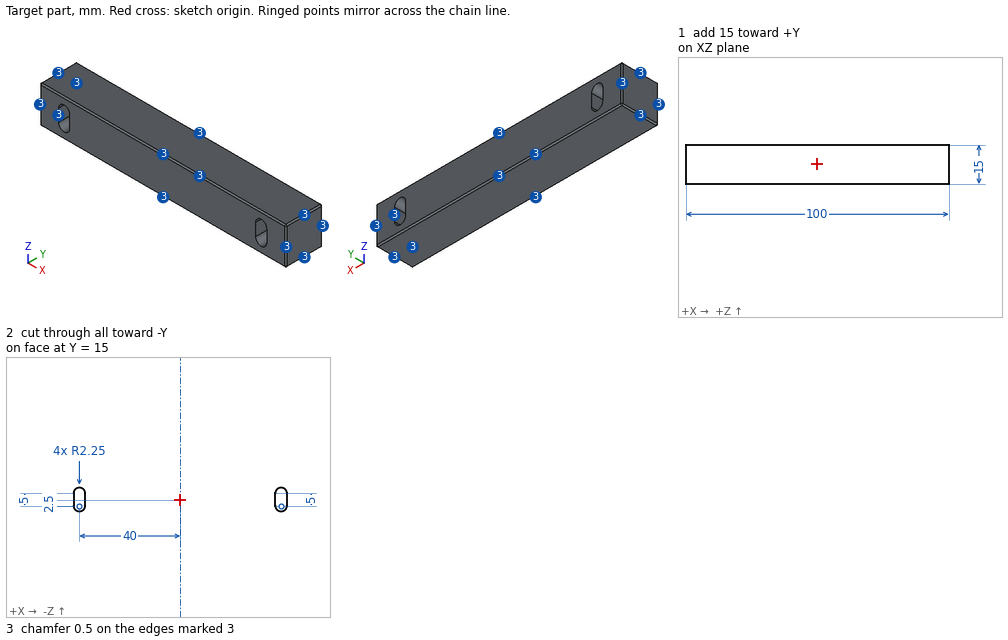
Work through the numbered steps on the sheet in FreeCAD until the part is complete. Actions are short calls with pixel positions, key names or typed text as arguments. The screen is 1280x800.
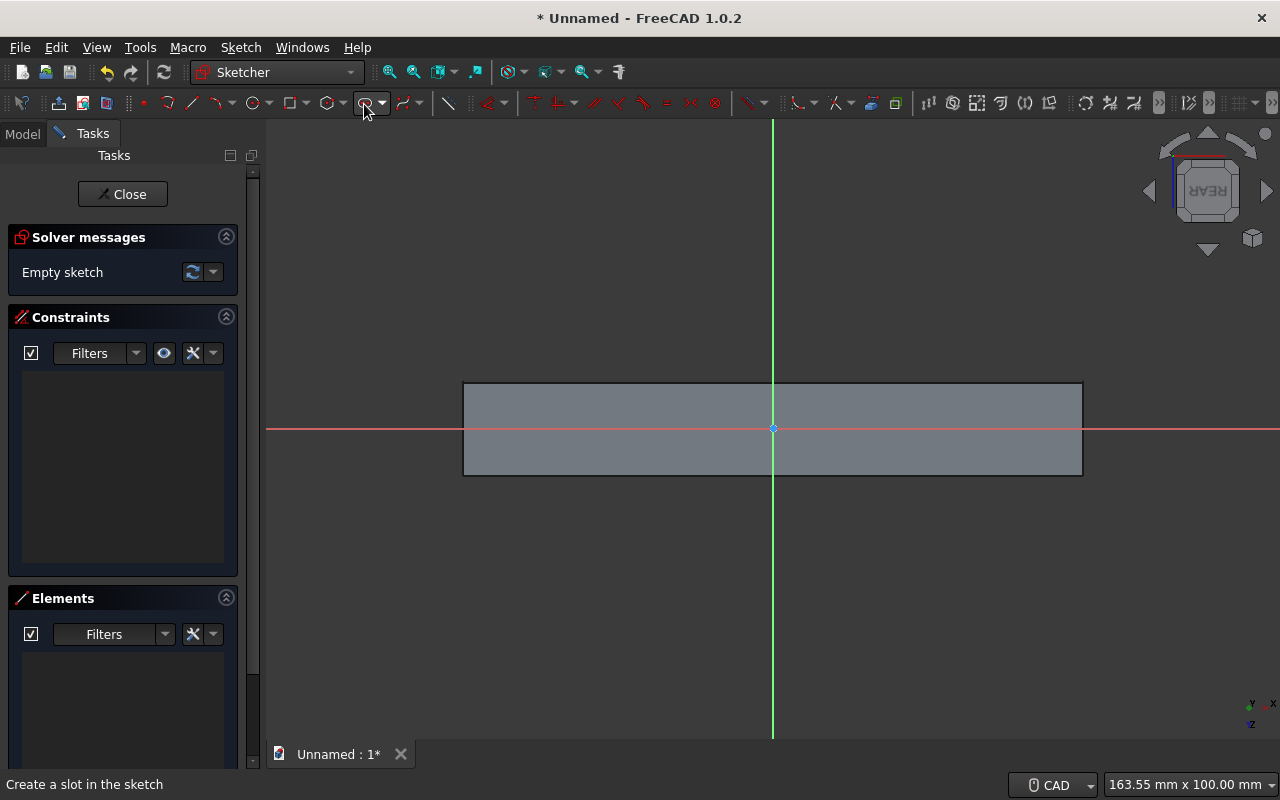
scroll(525, 445, up, 3)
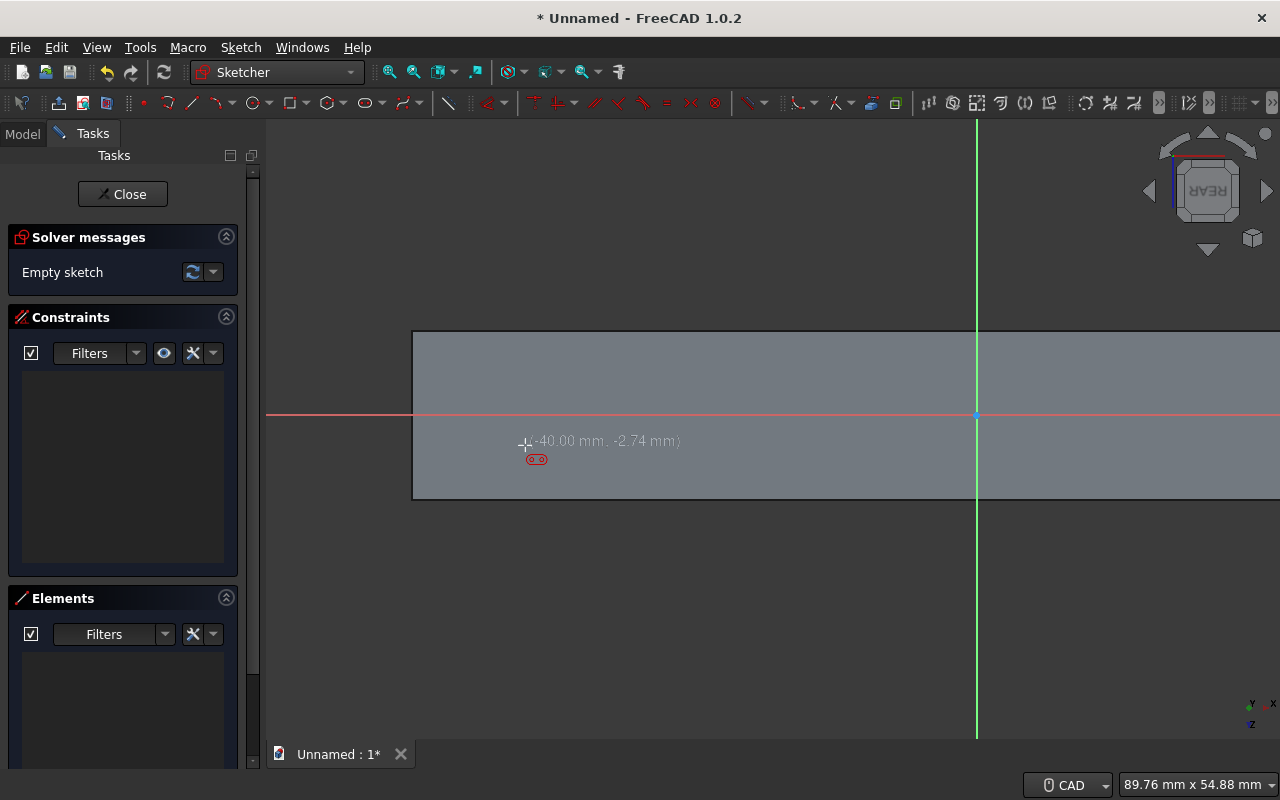
click(525, 444)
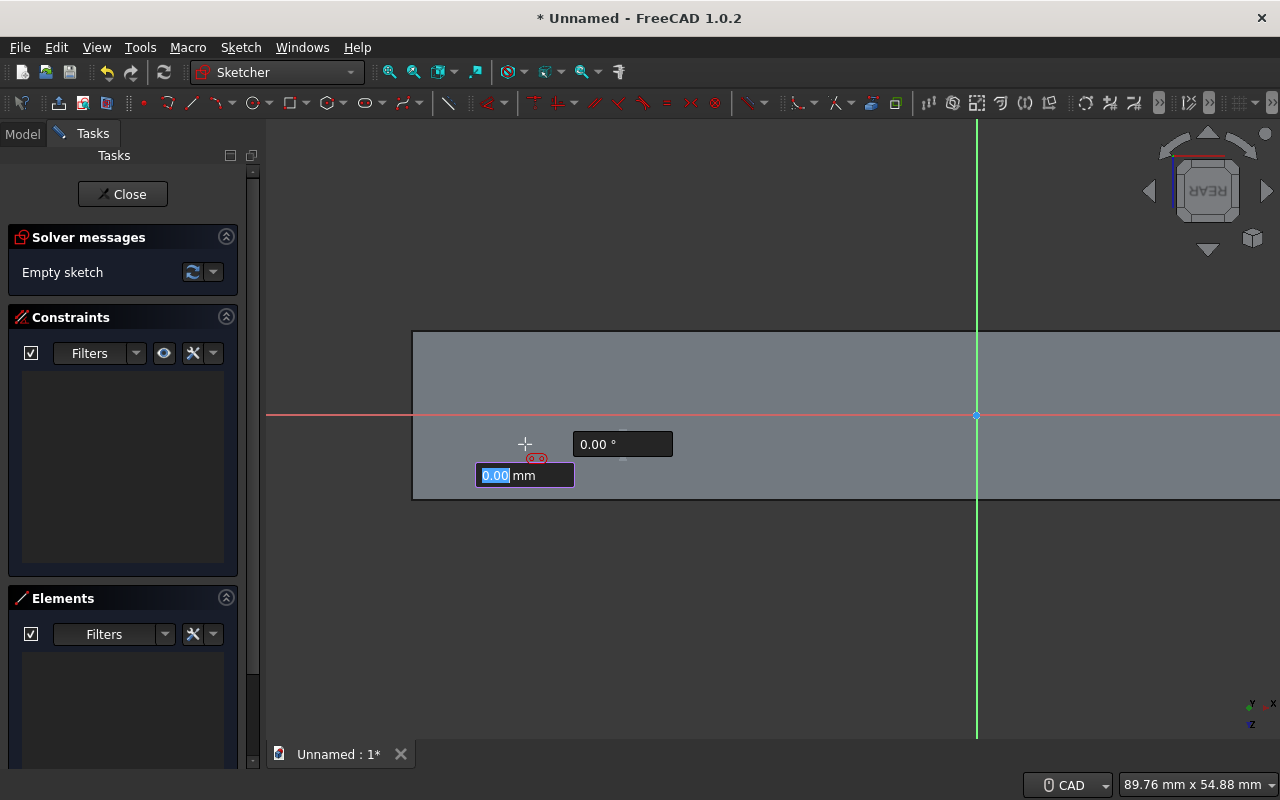
click(525, 387)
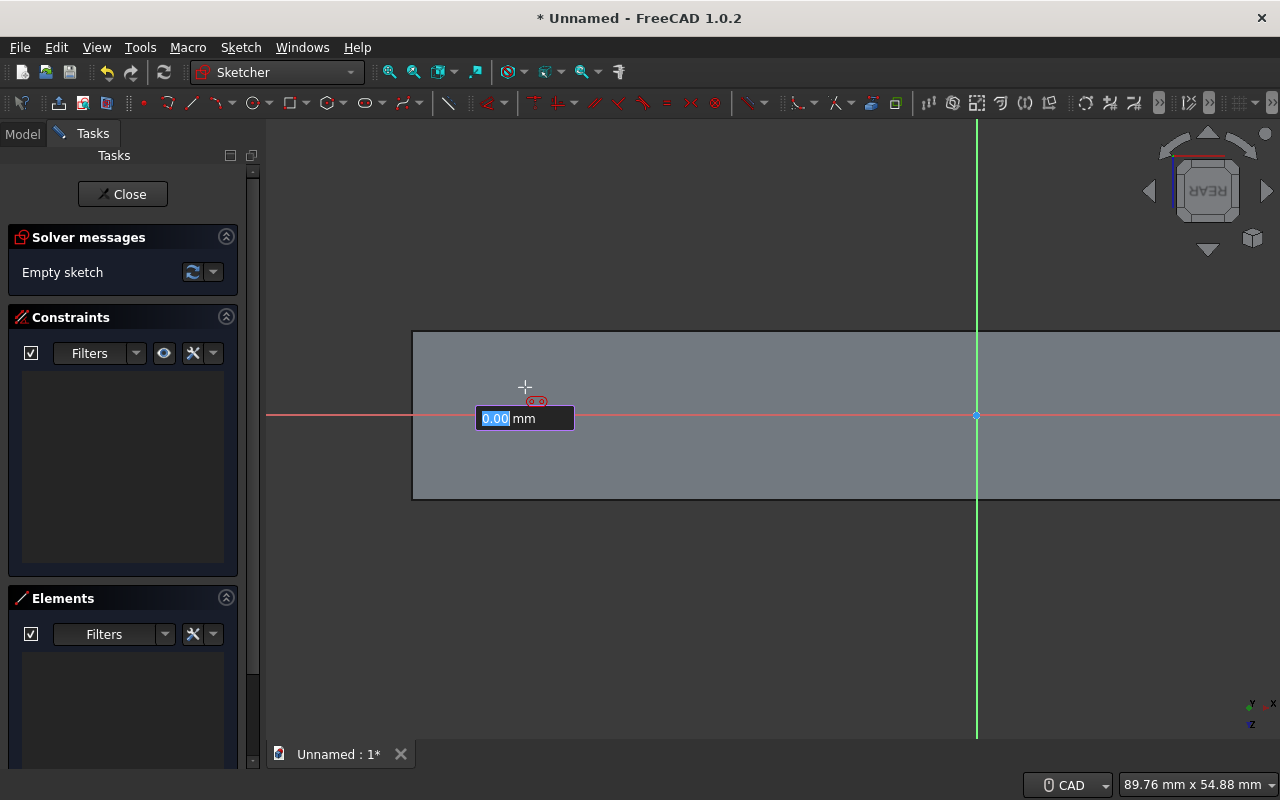
scroll(499, 407, up, 4)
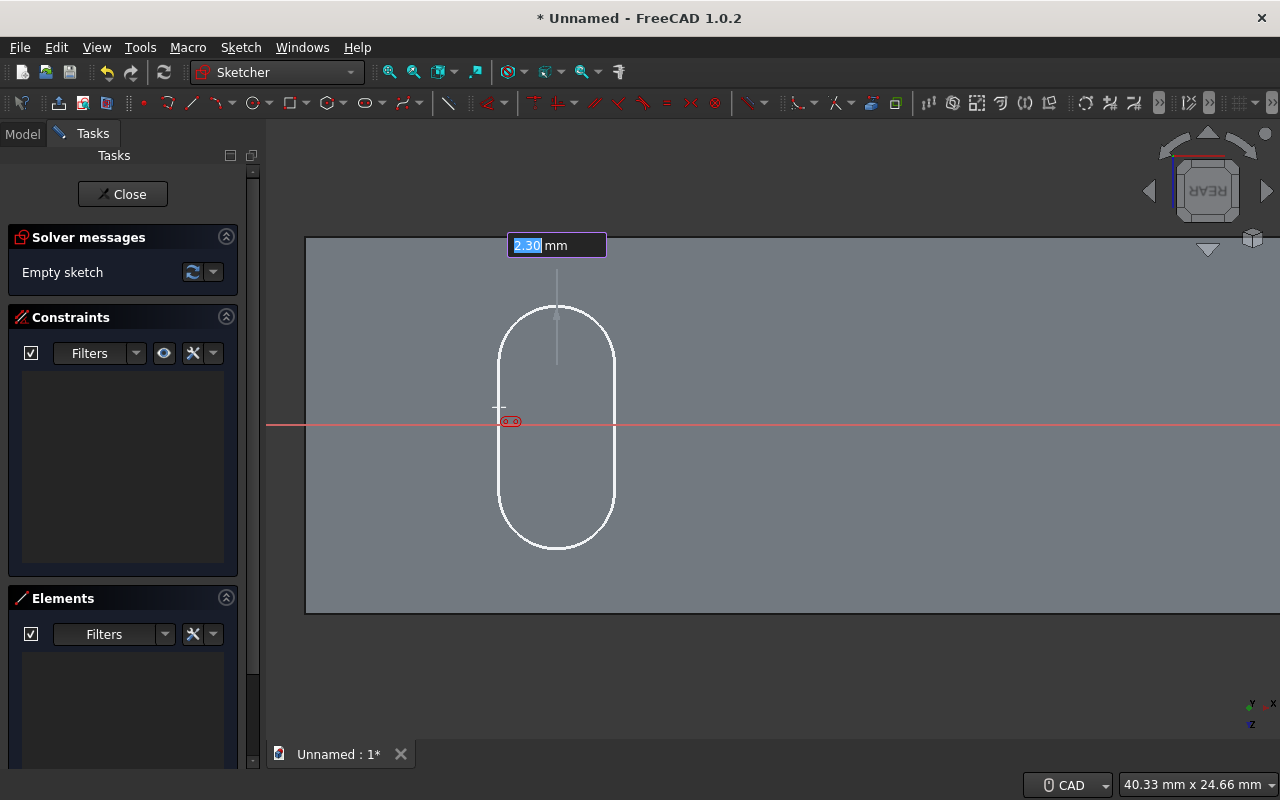
click(500, 406)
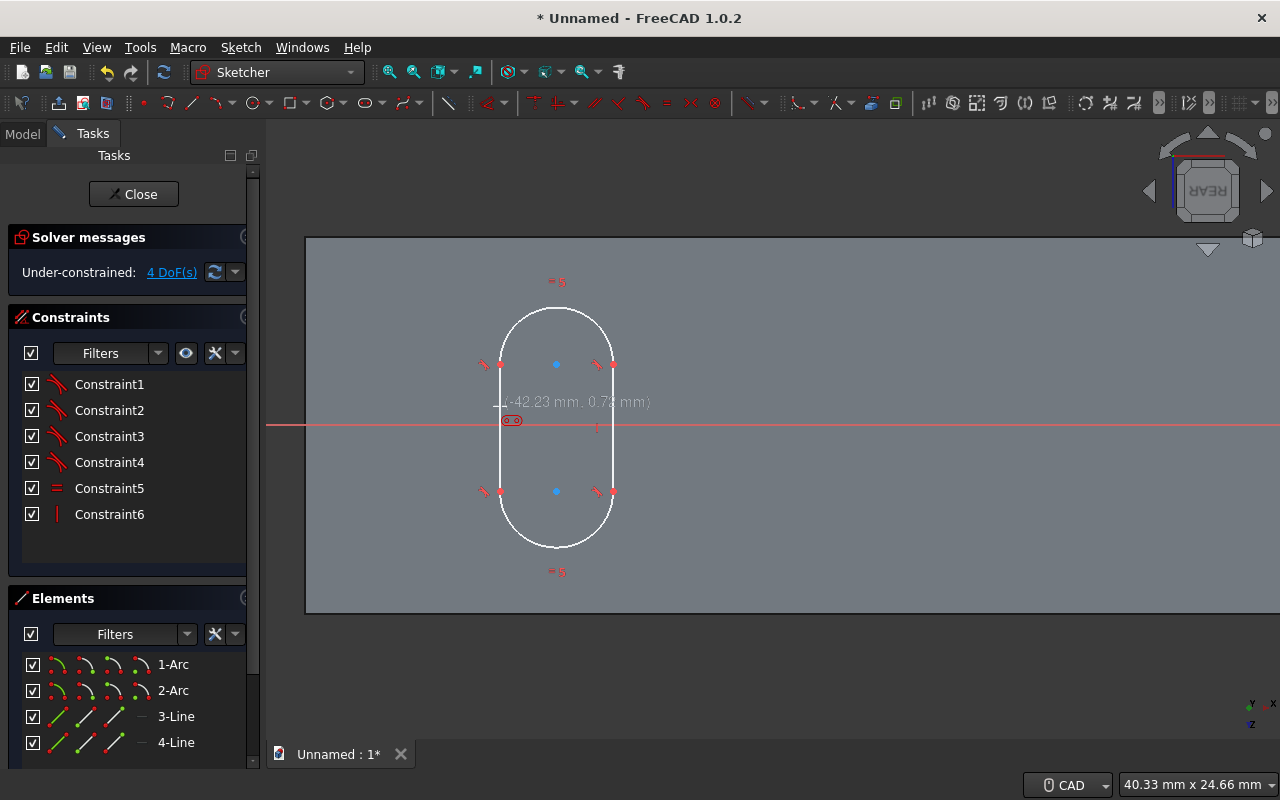
scroll(335, 431, down, 6)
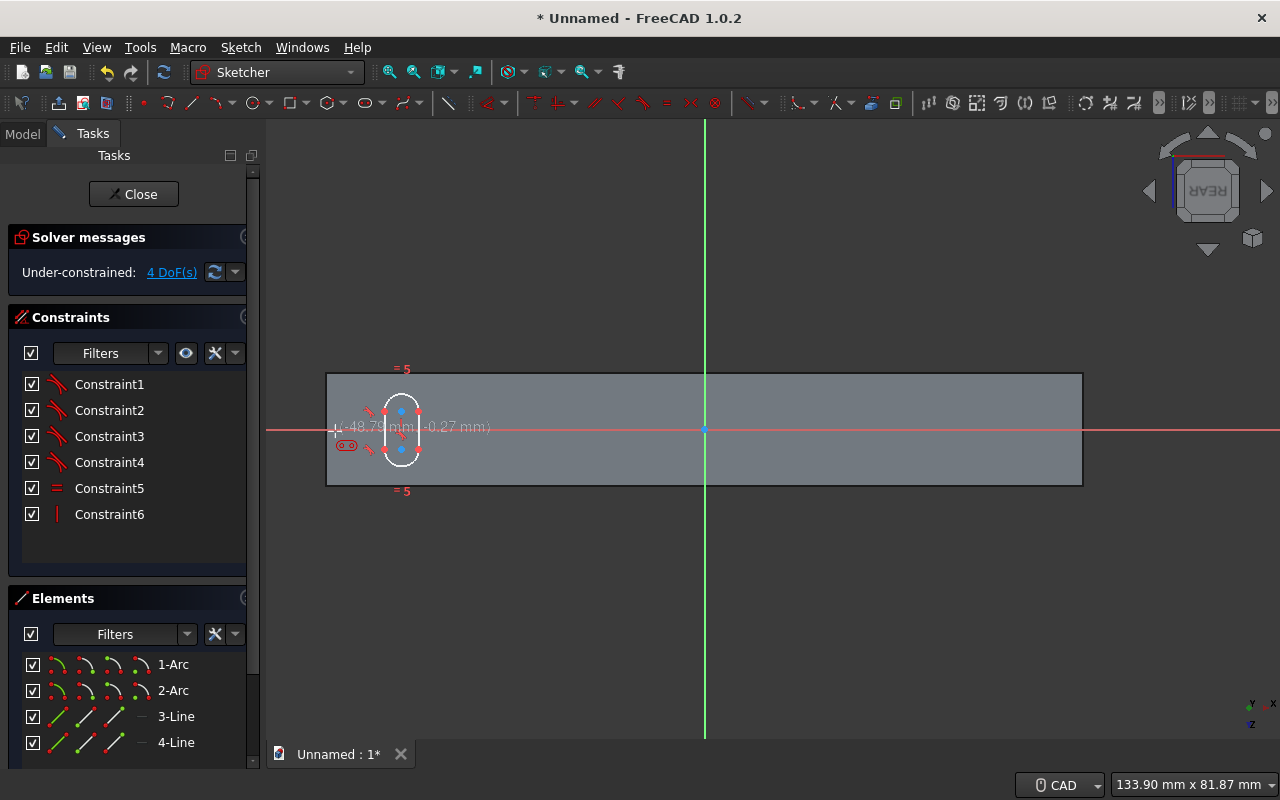
scroll(1007, 449, up, 2)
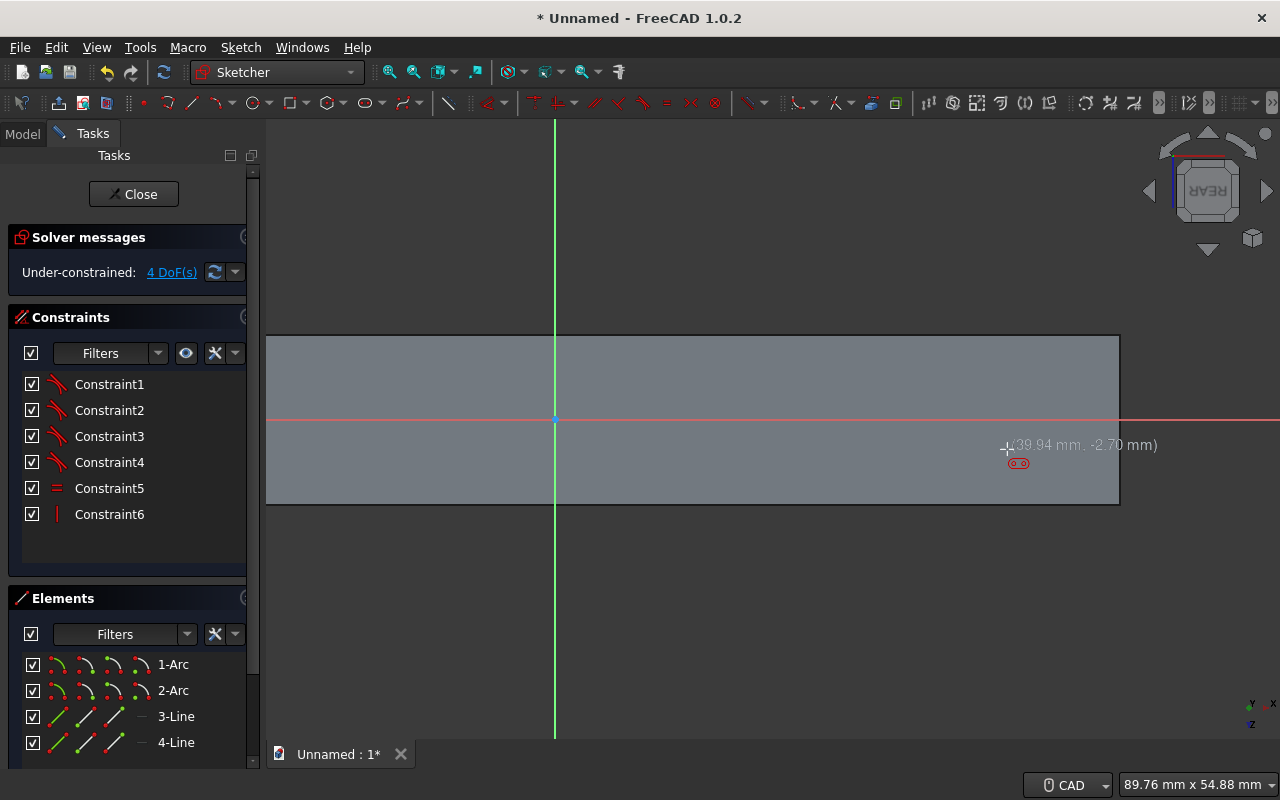
click(1007, 448)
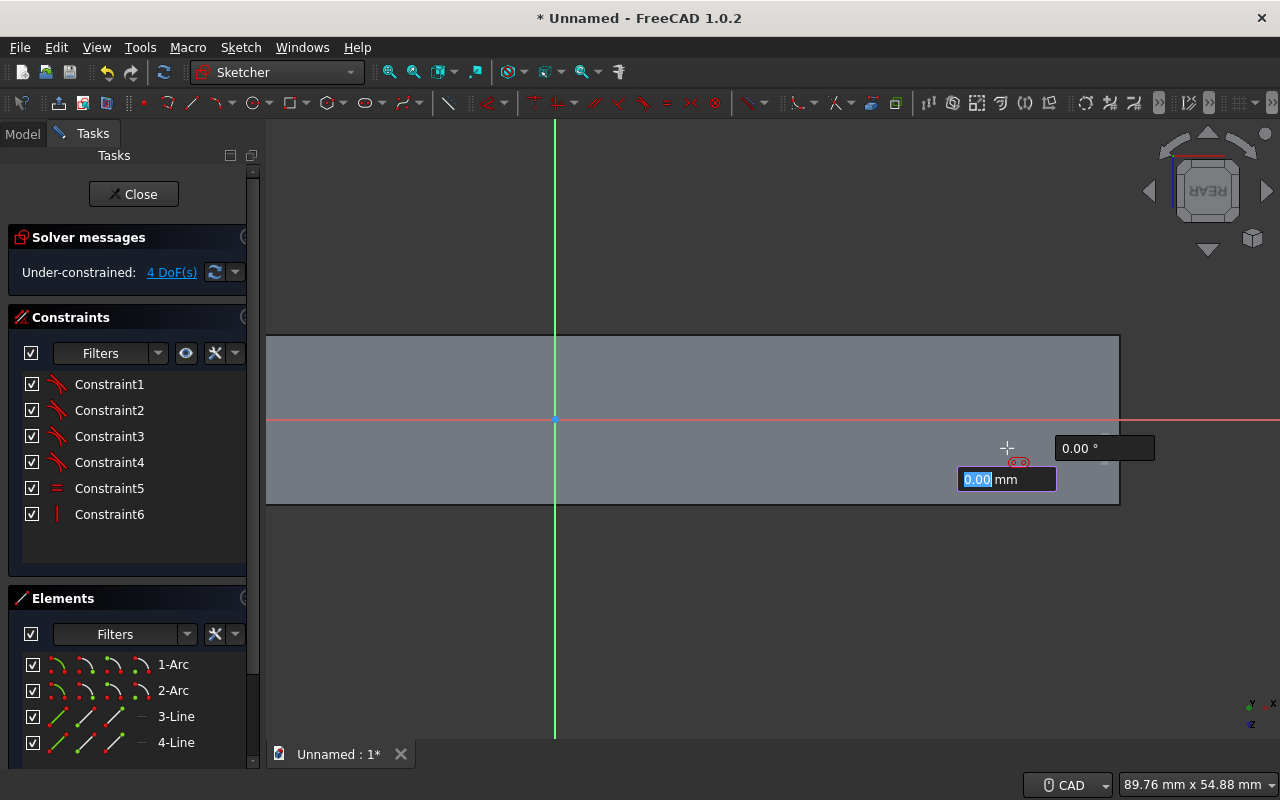
click(1007, 392)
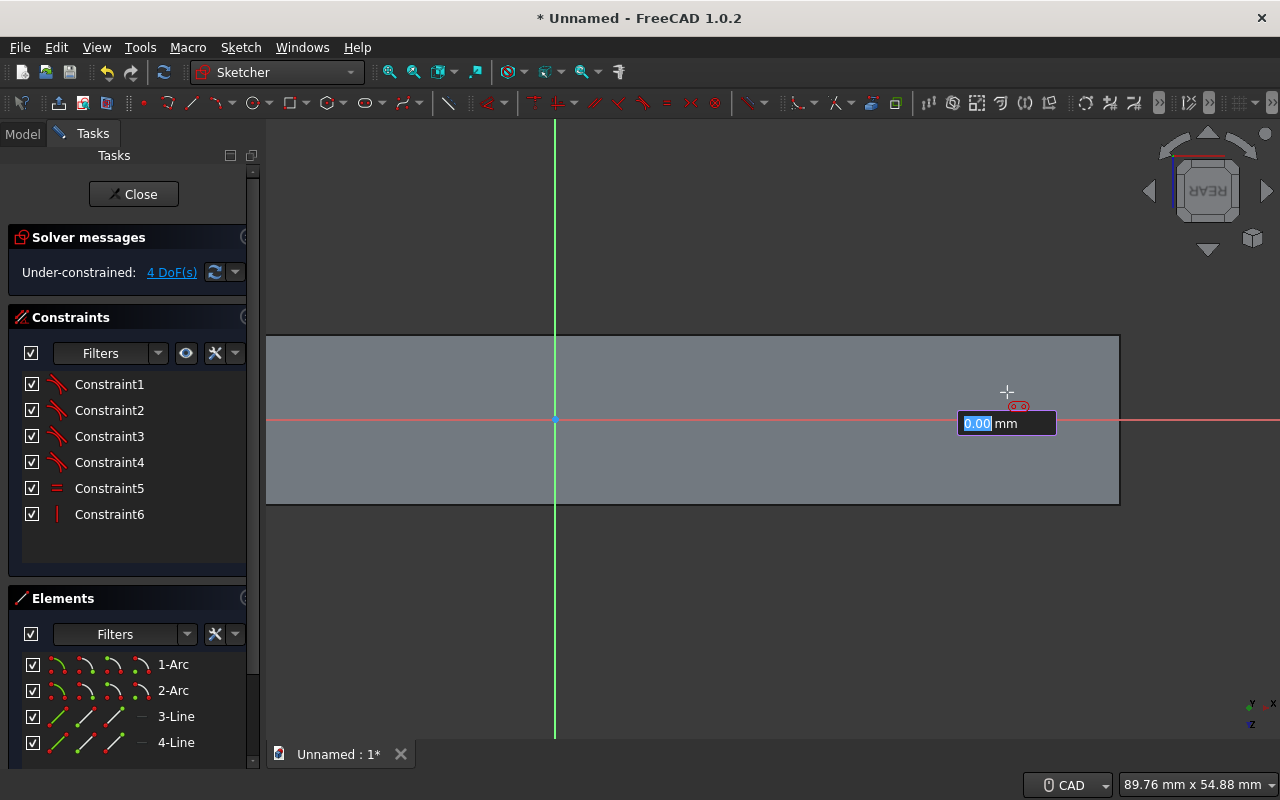
scroll(982, 411, up, 4)